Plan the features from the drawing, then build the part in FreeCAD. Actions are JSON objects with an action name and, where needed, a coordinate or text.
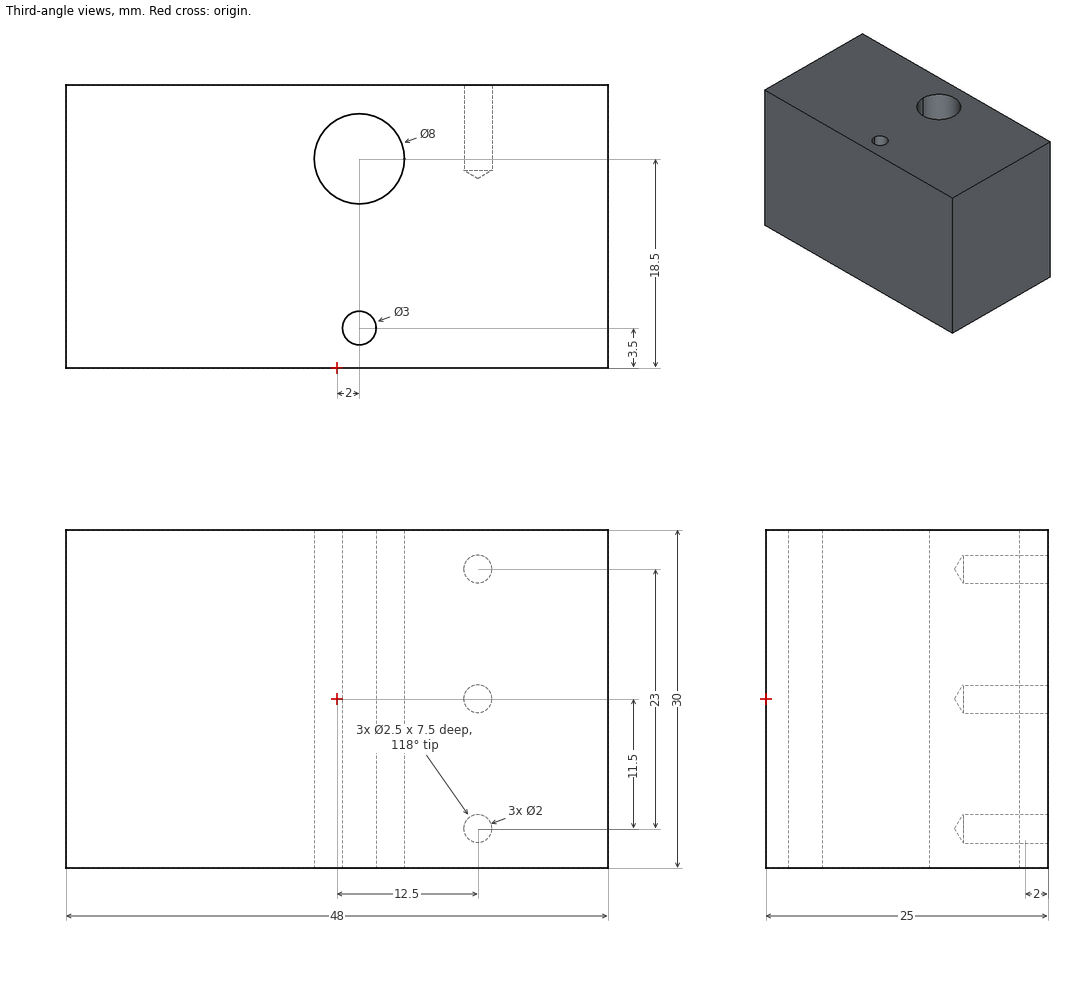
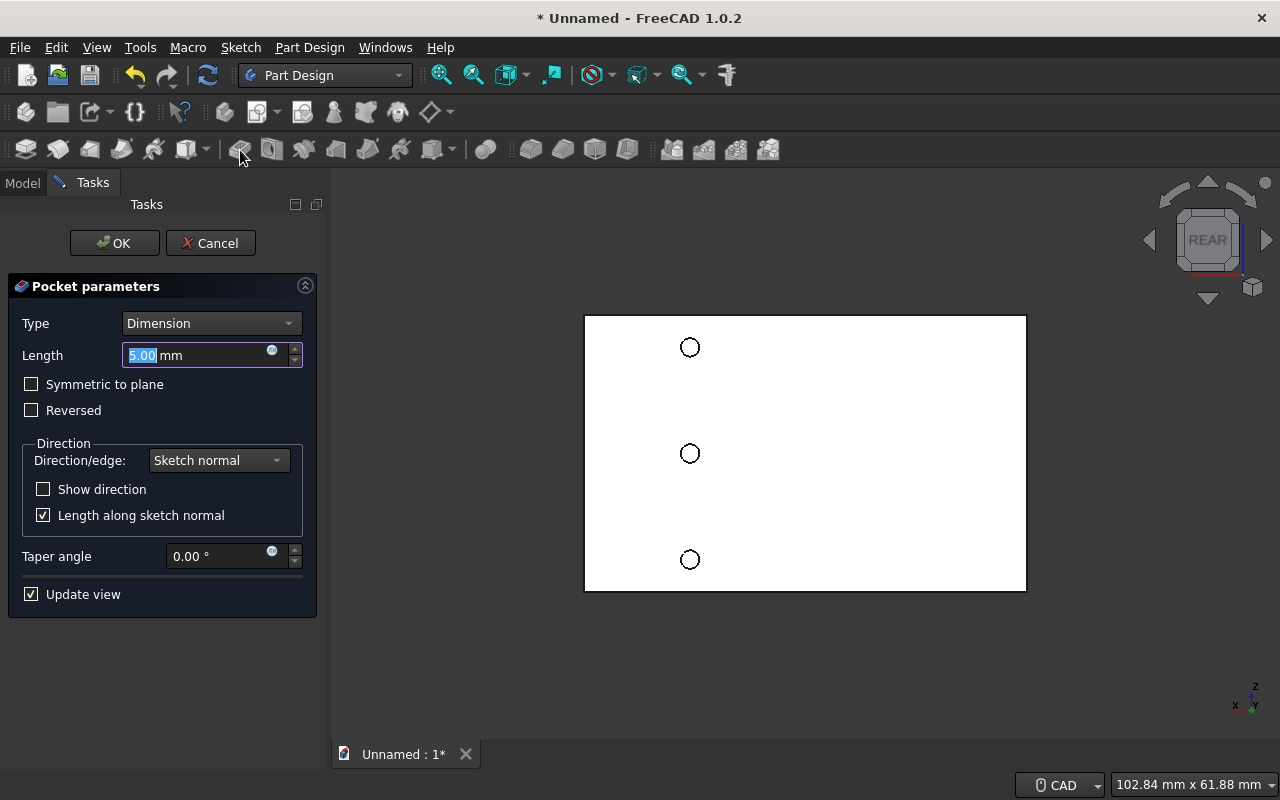
{"action": "type", "text": "2"}
{"action": "key", "text": "Tab"}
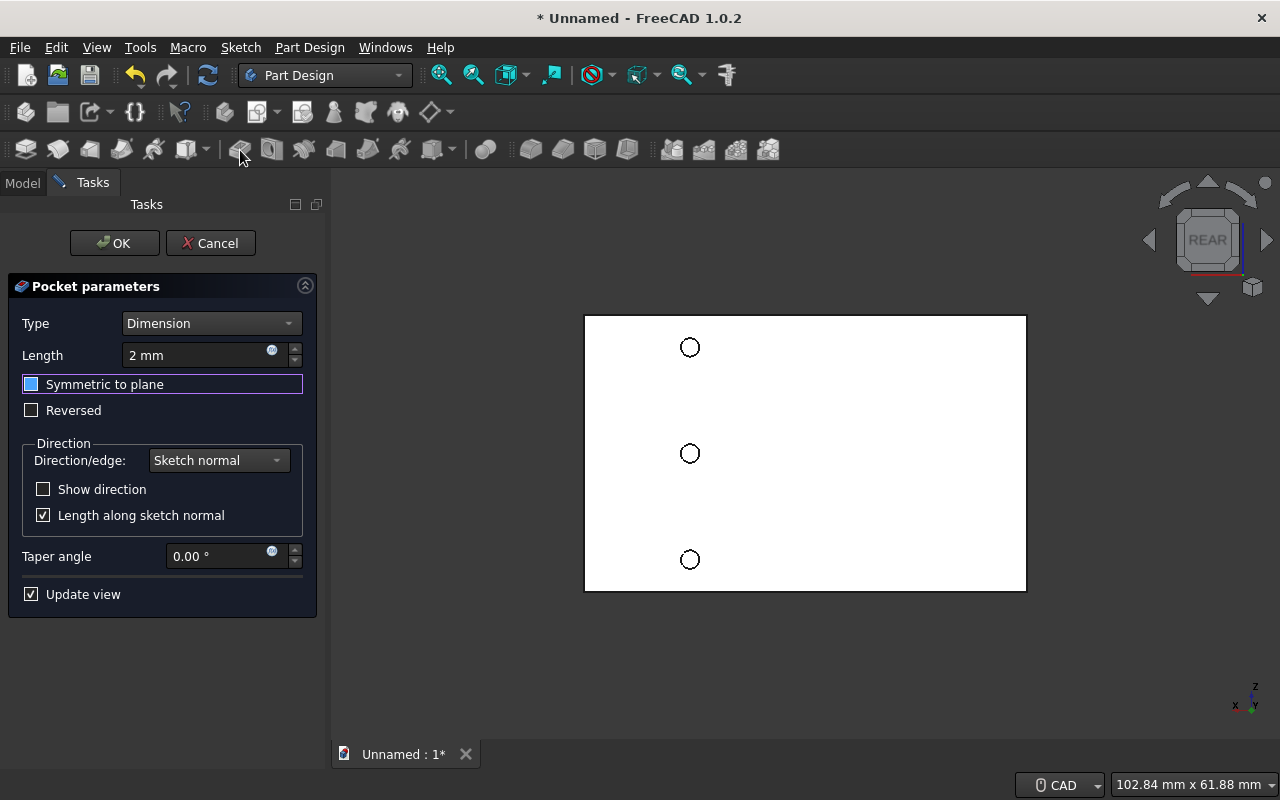
{"action": "left_click", "coordinate": [115, 243]}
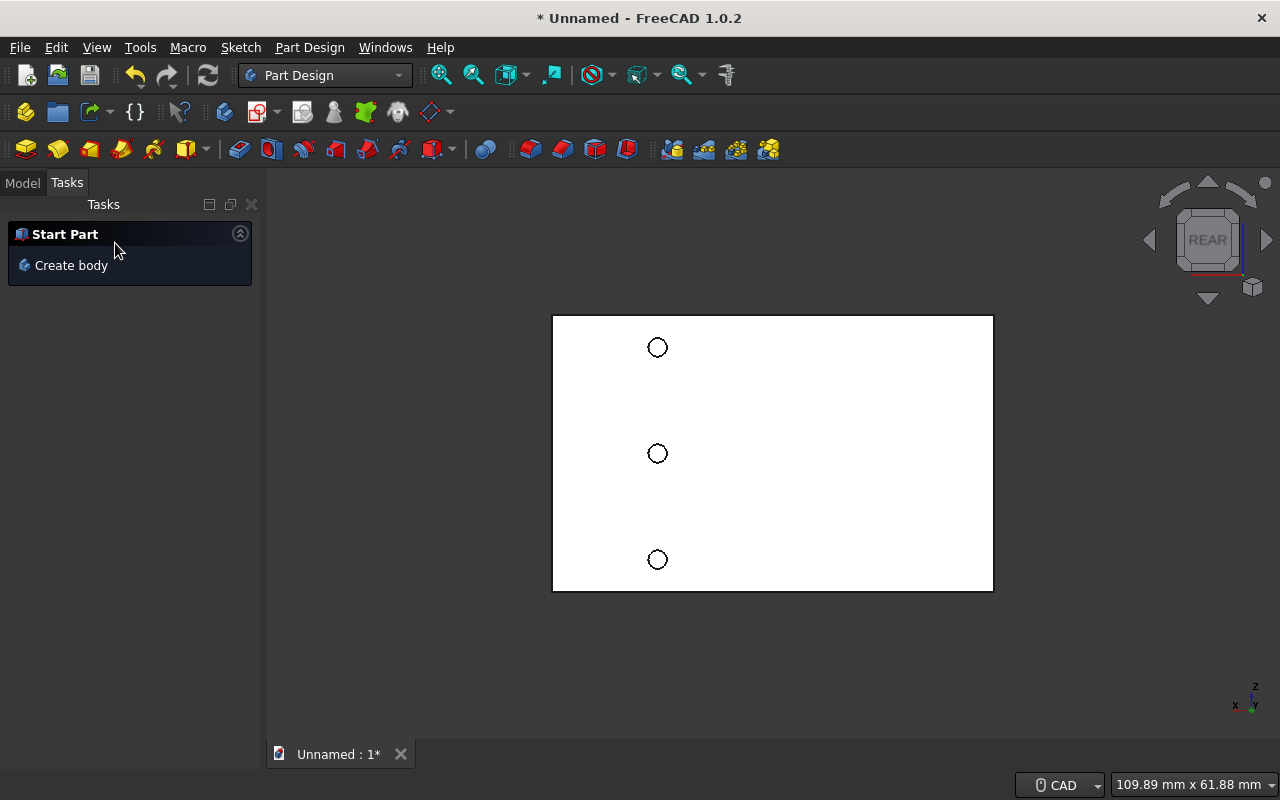
{"action": "left_click", "coordinate": [836, 453]}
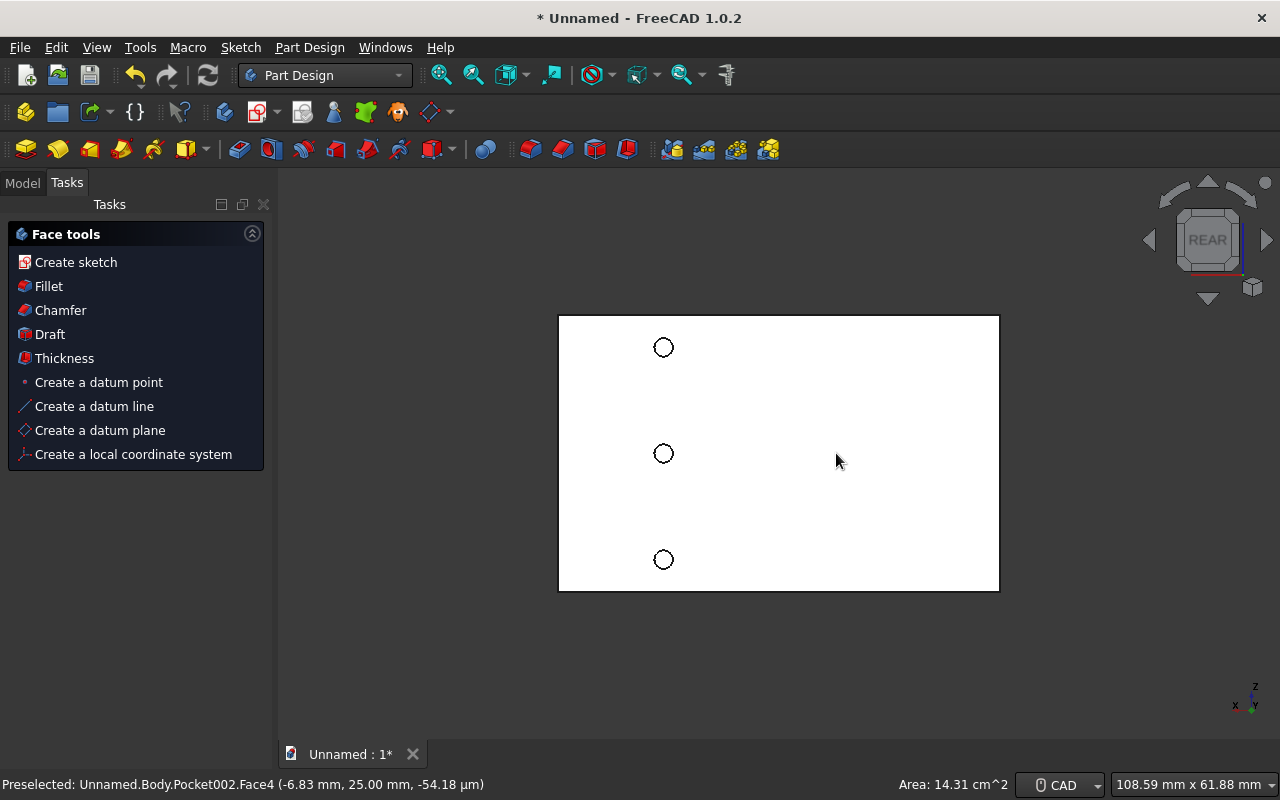
{"action": "left_click", "coordinate": [258, 112]}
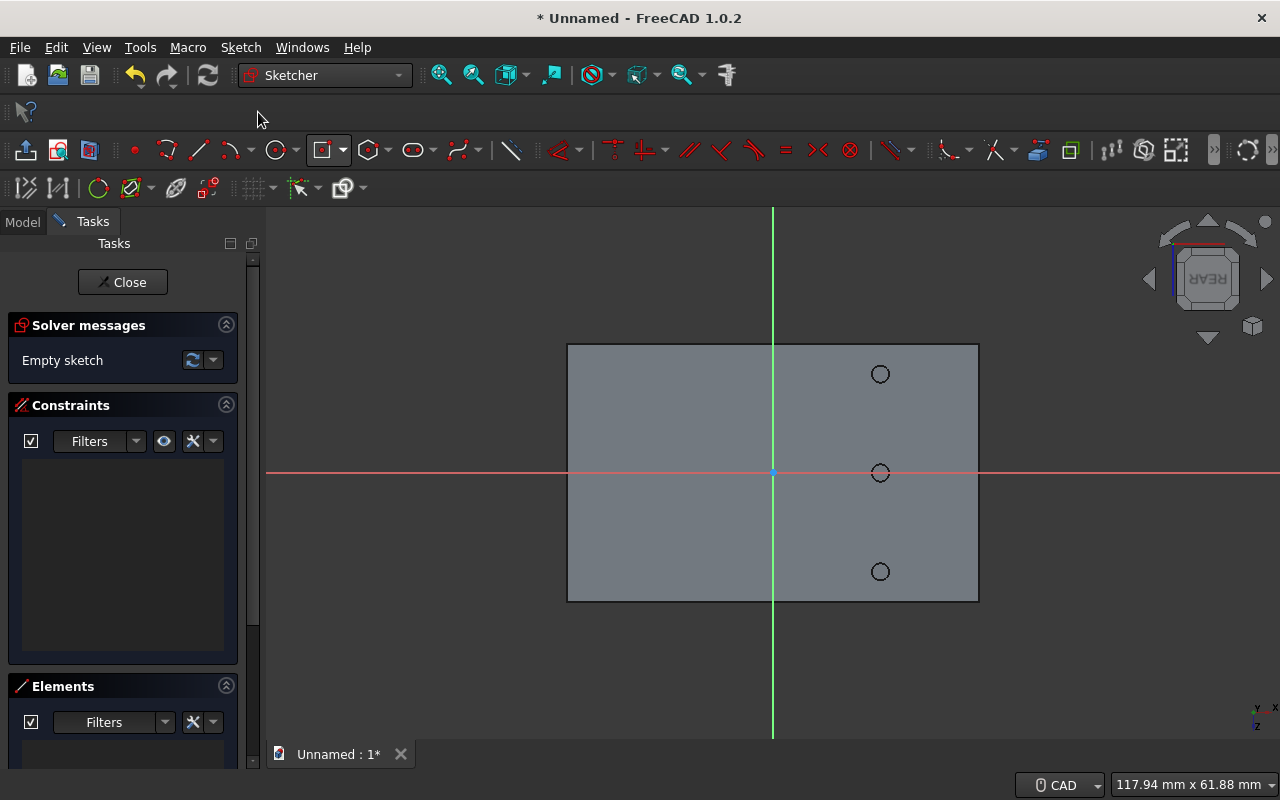
{"action": "scroll", "coordinate": [1092, 473], "scroll_direction": "up", "scroll_amount": 2}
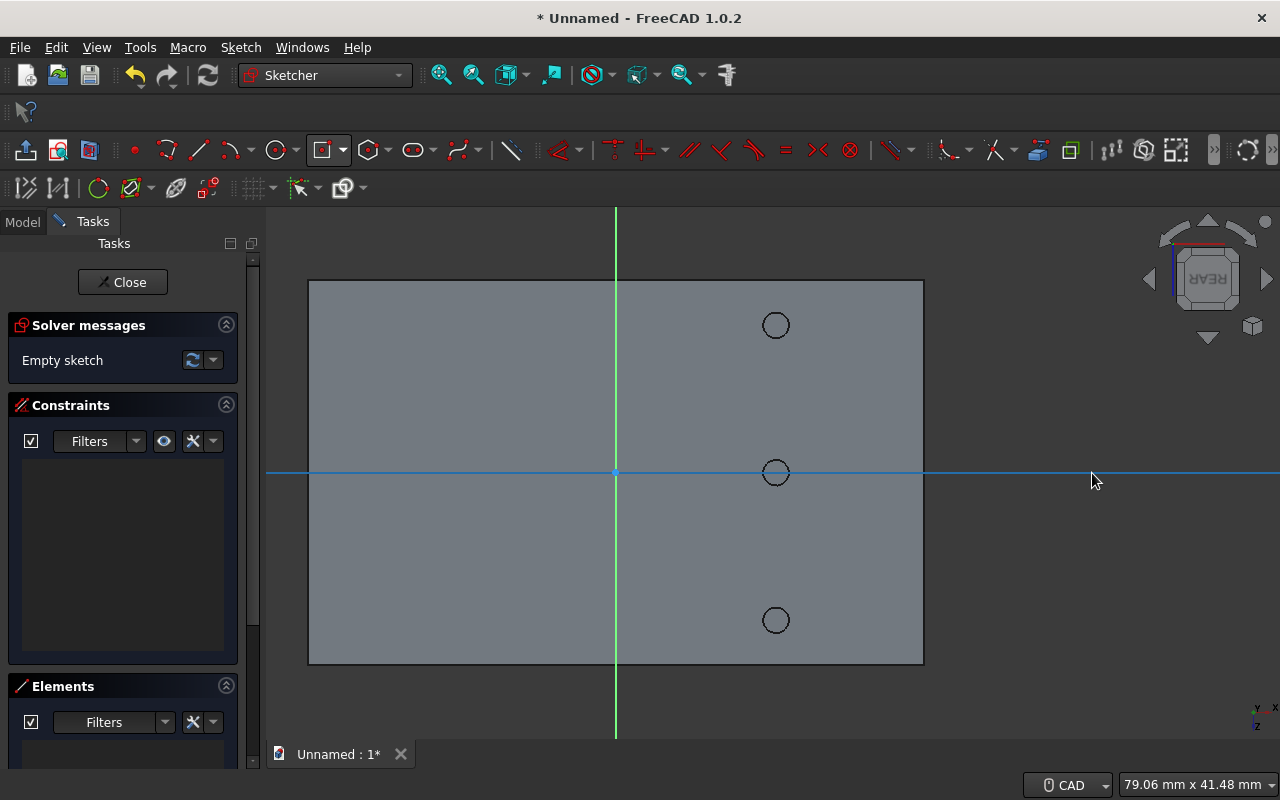
{"action": "key", "text": "g c"}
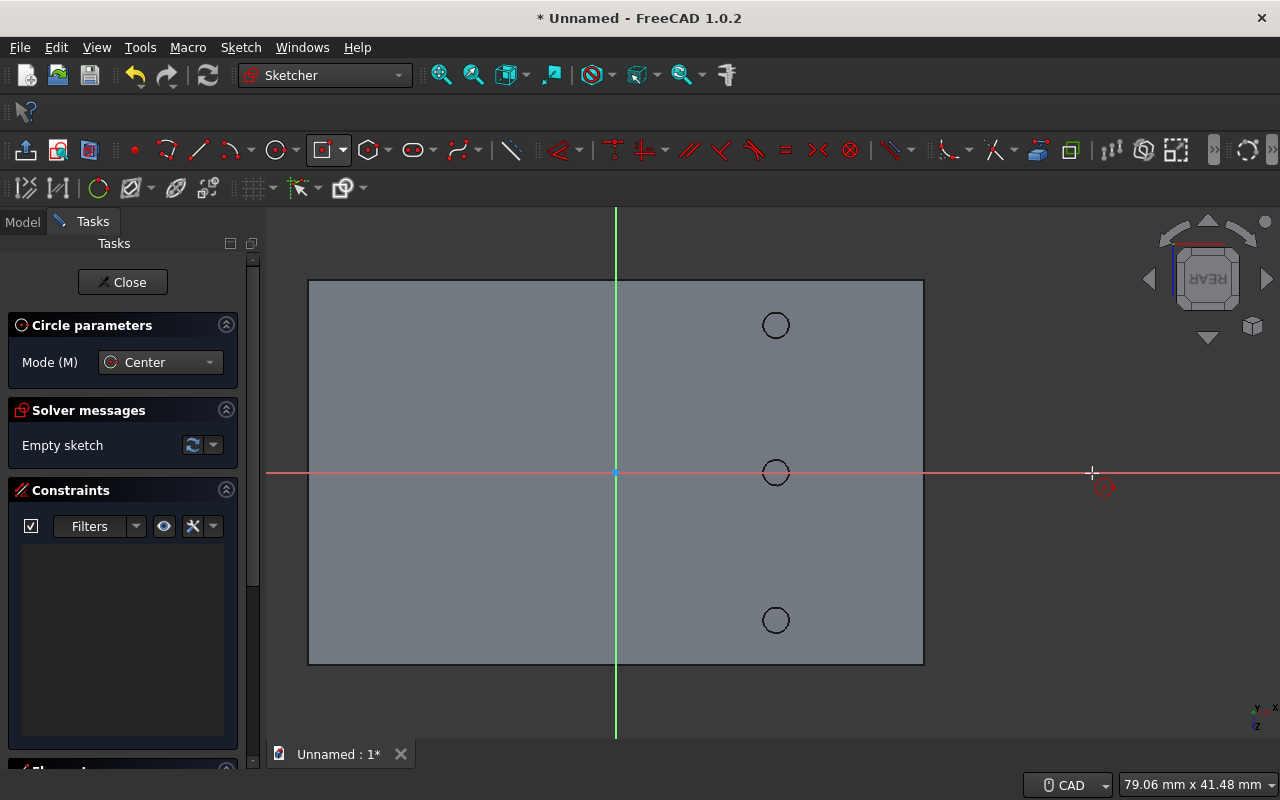
{"action": "scroll", "coordinate": [776, 325], "scroll_direction": "up", "scroll_amount": 2}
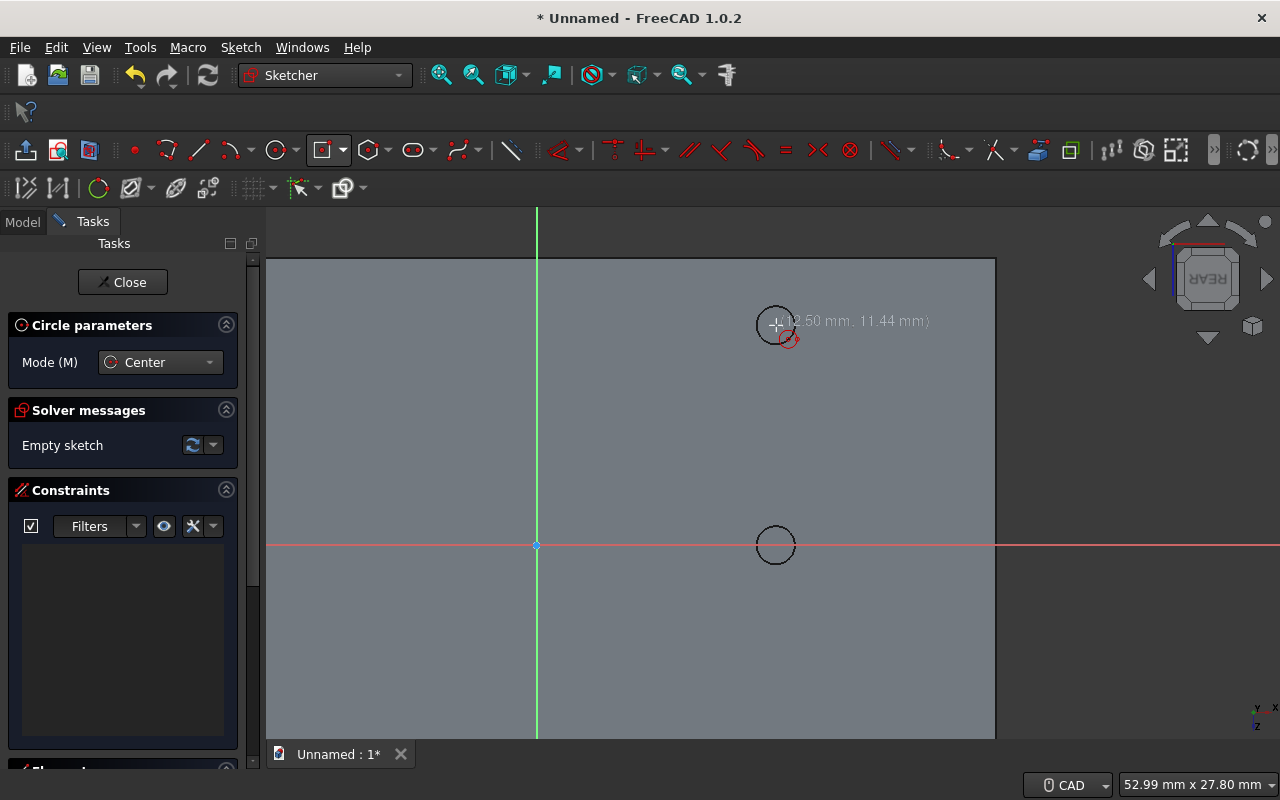
{"action": "left_click", "coordinate": [776, 325]}
{"action": "left_click", "coordinate": [793, 308]}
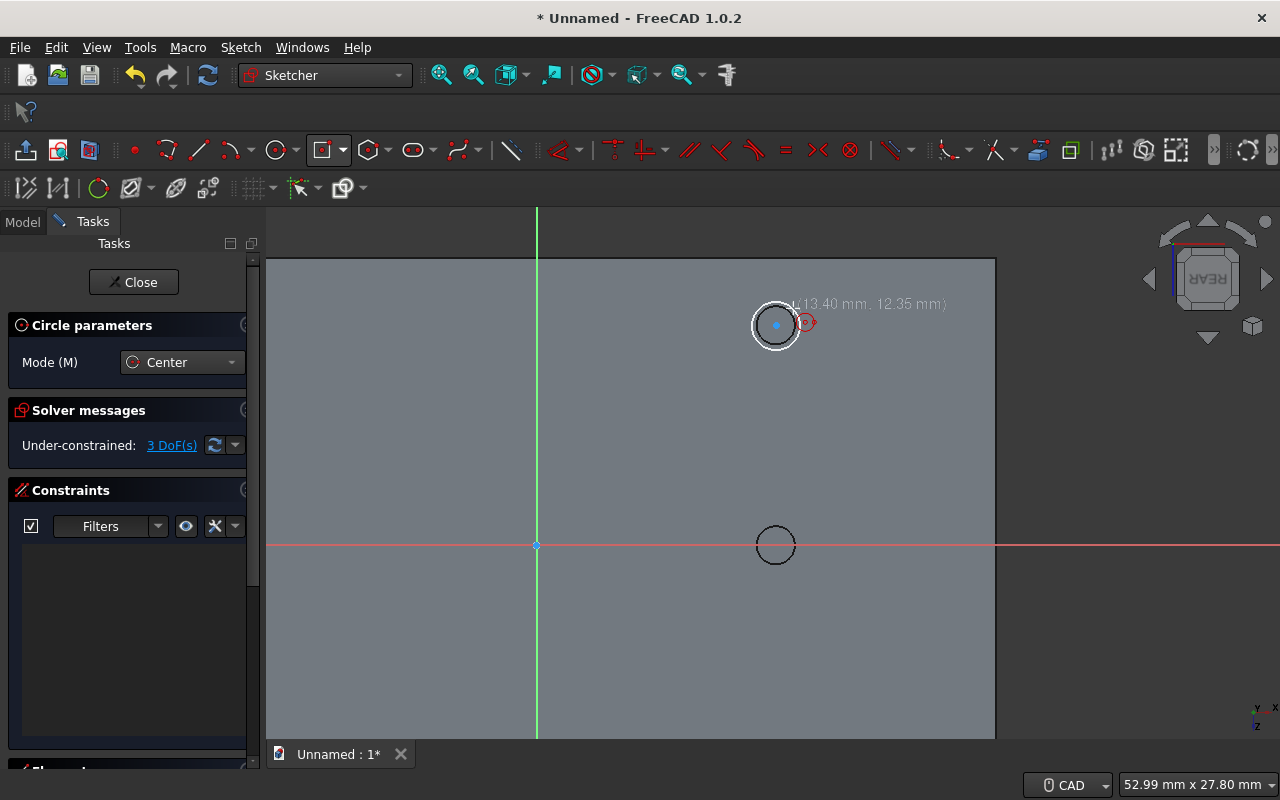
{"action": "left_click", "coordinate": [776, 545]}
{"action": "left_click", "coordinate": [793, 528]}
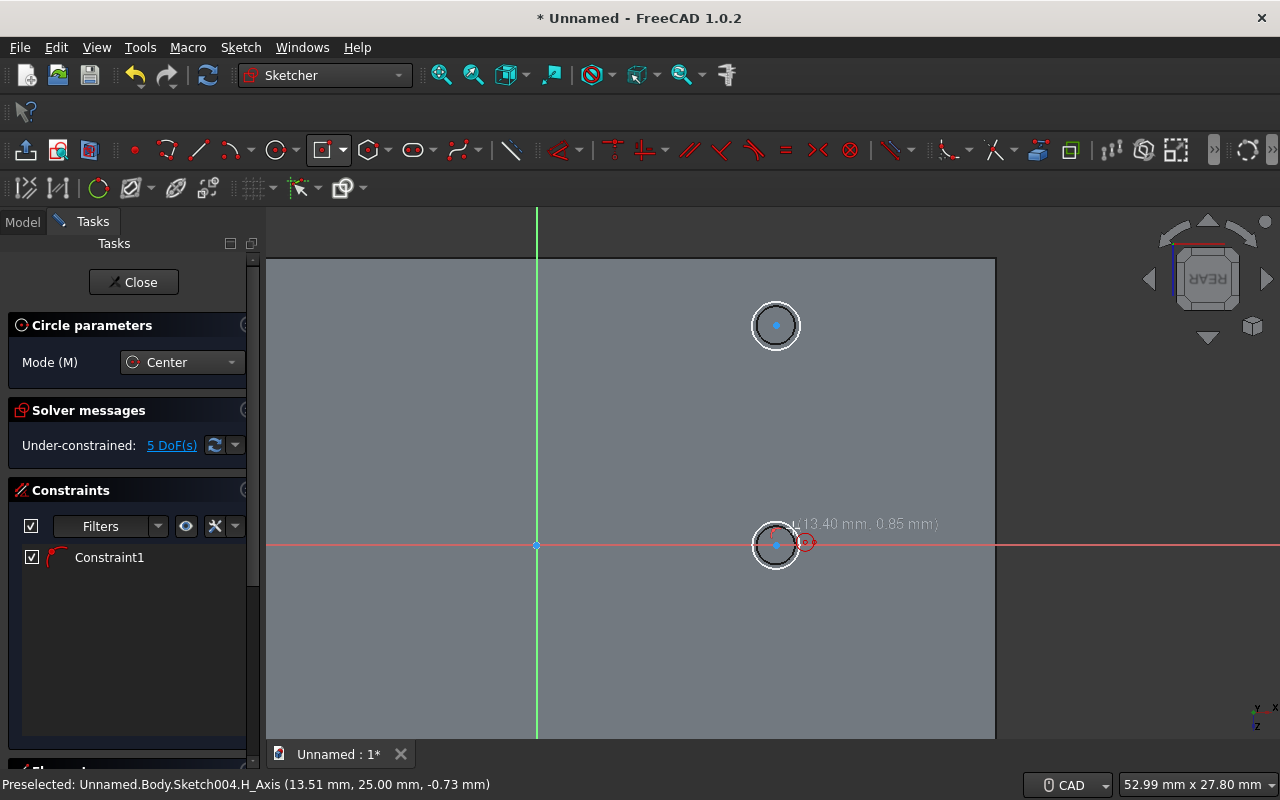
{"action": "scroll", "coordinate": [778, 326], "scroll_direction": "down", "scroll_amount": 2}